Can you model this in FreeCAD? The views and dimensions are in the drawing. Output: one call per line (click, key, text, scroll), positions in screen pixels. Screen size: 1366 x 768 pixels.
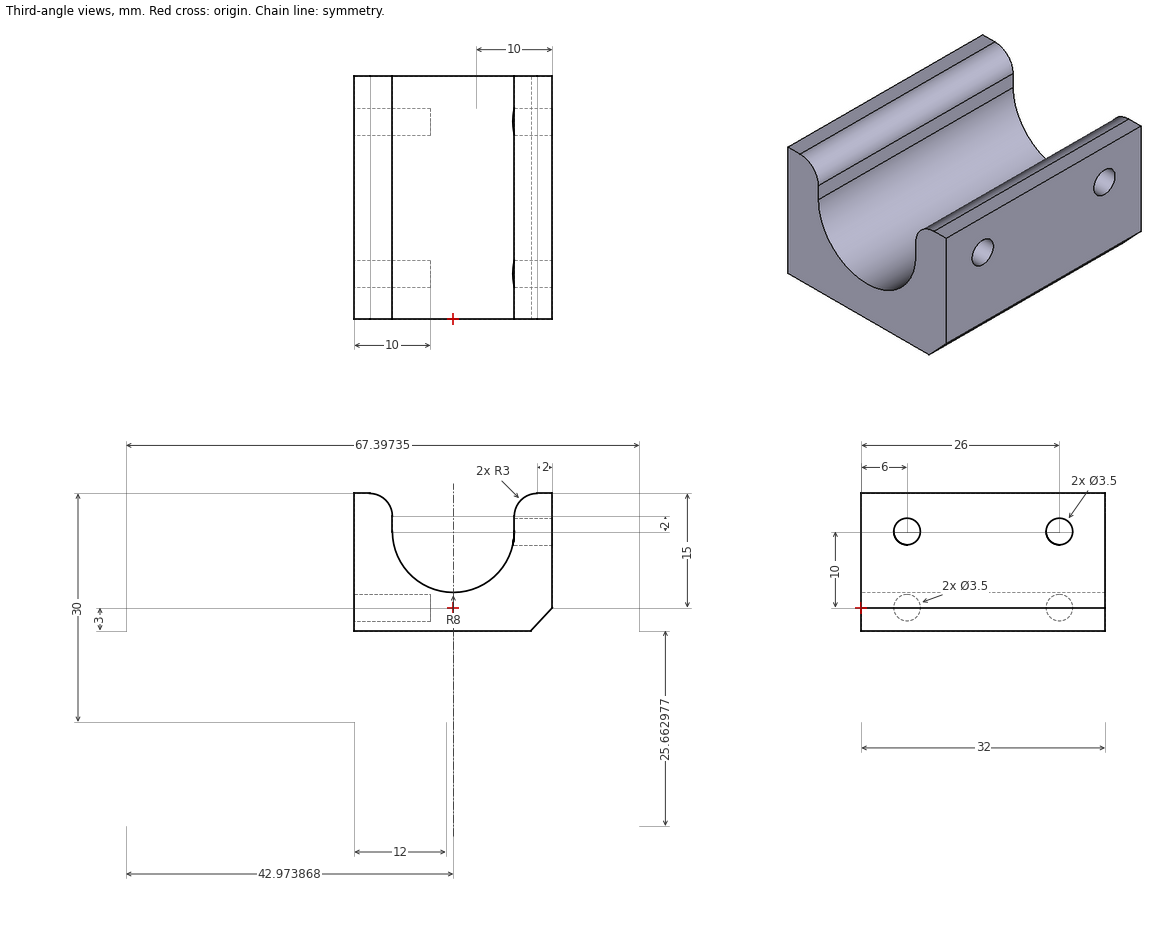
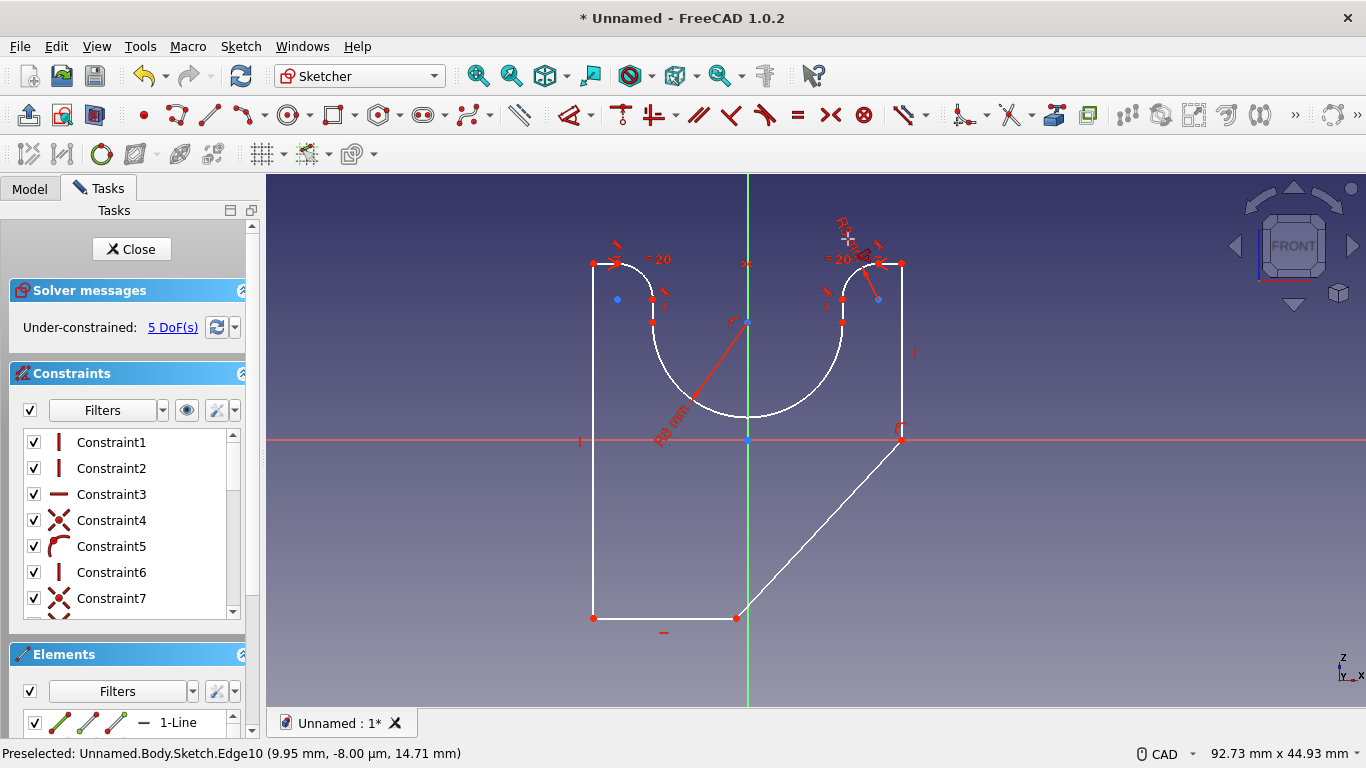
scroll(653, 309, up, 3)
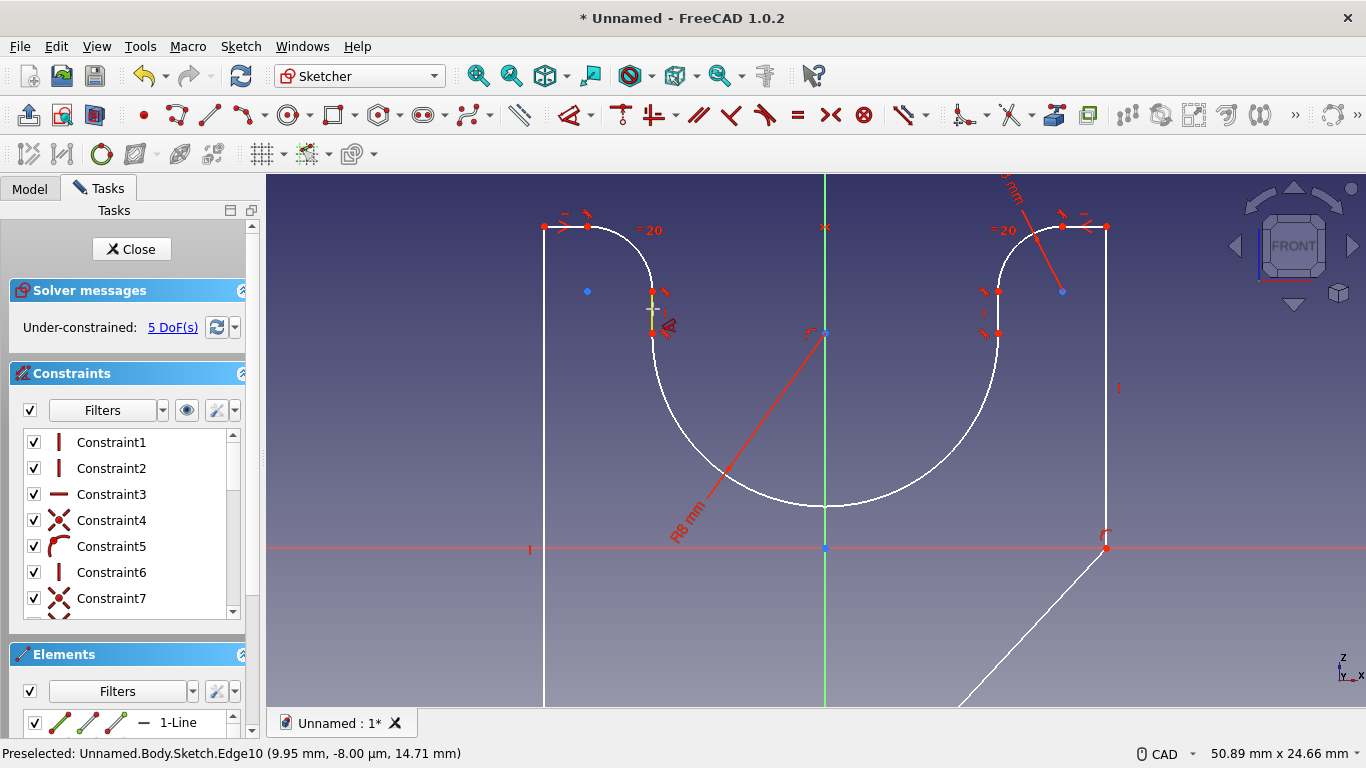
click(652, 308)
click(618, 313)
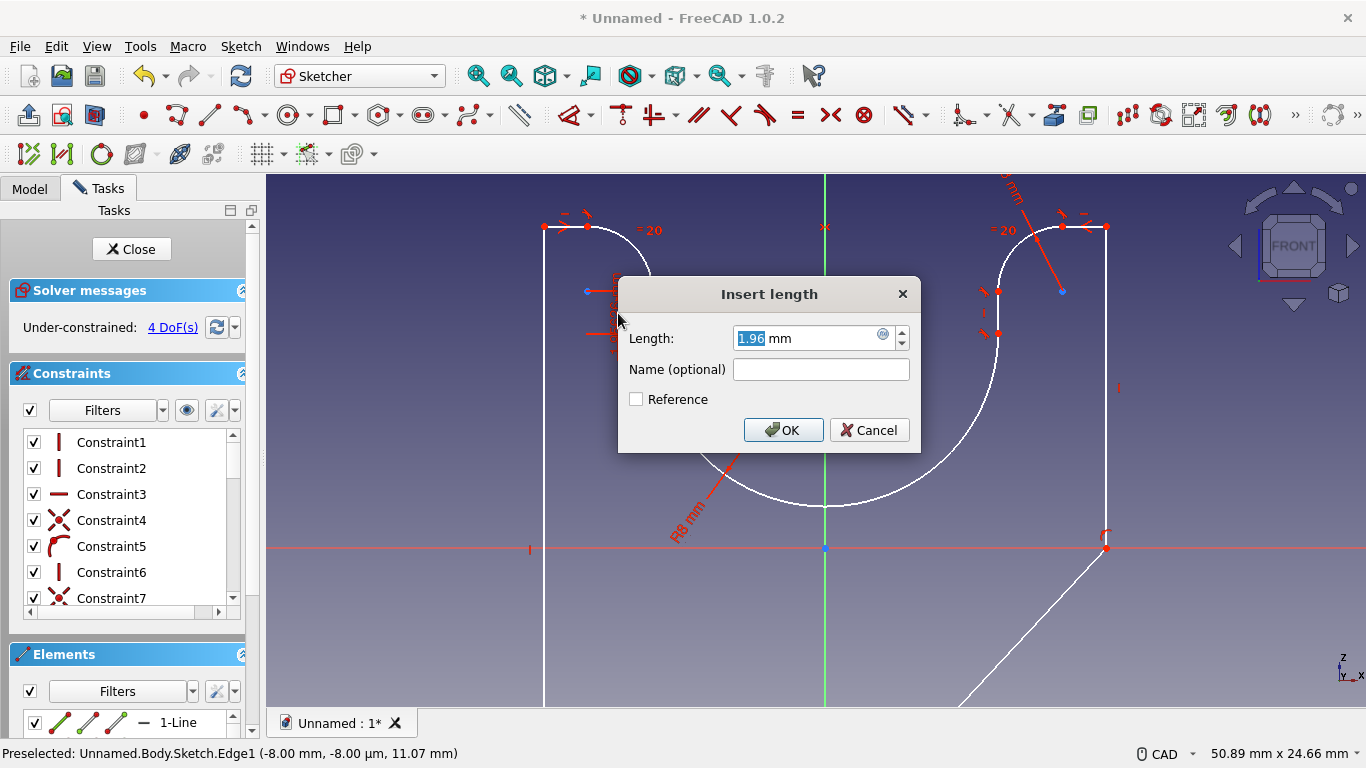
text(2)
key(Return)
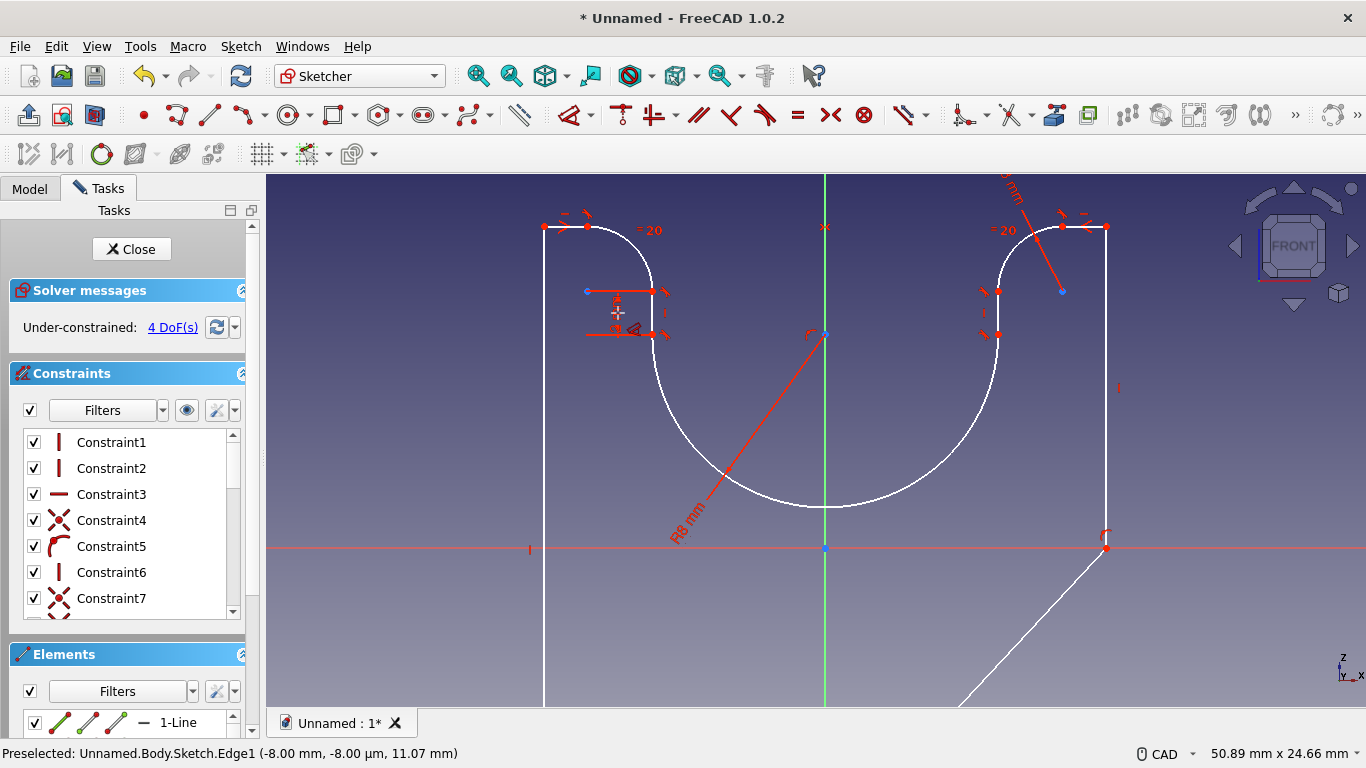
click(1076, 227)
click(1085, 261)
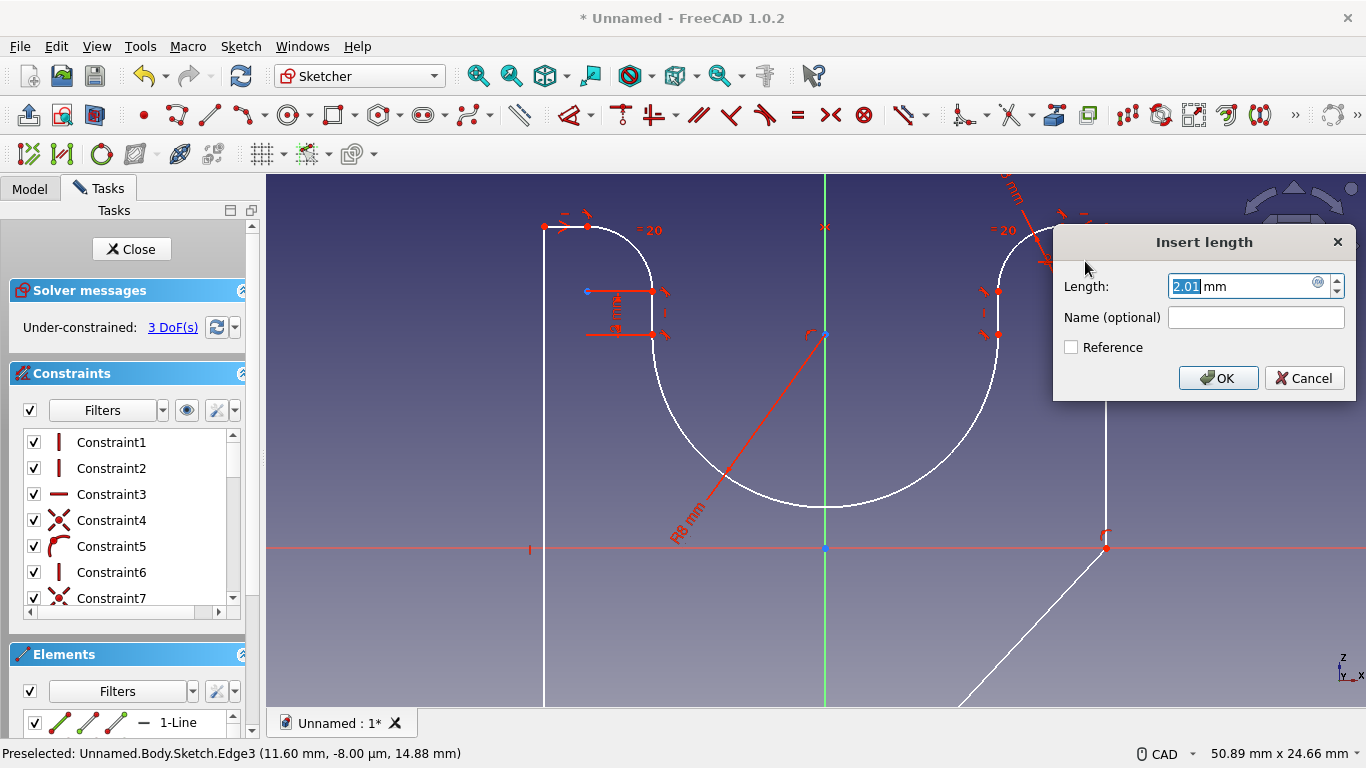
text(2)
key(Return)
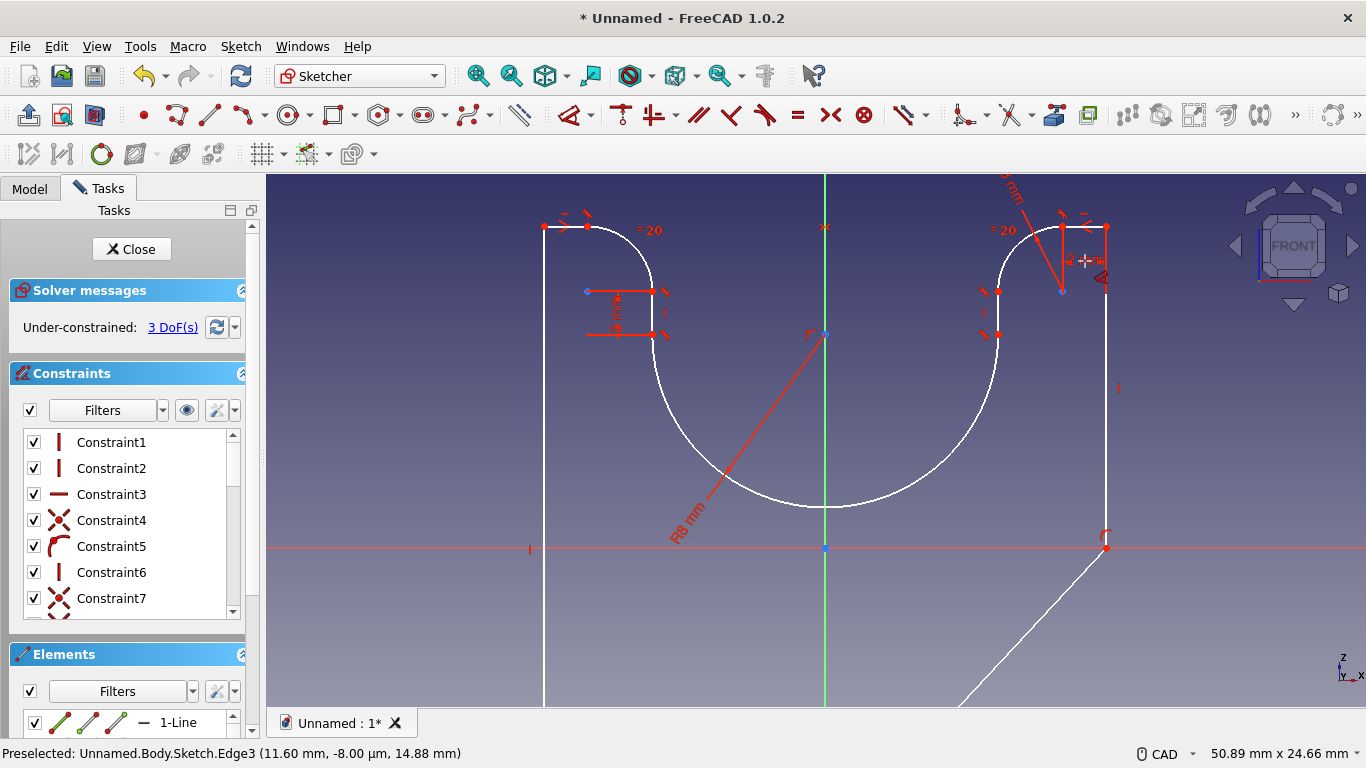
click(1106, 323)
click(1140, 387)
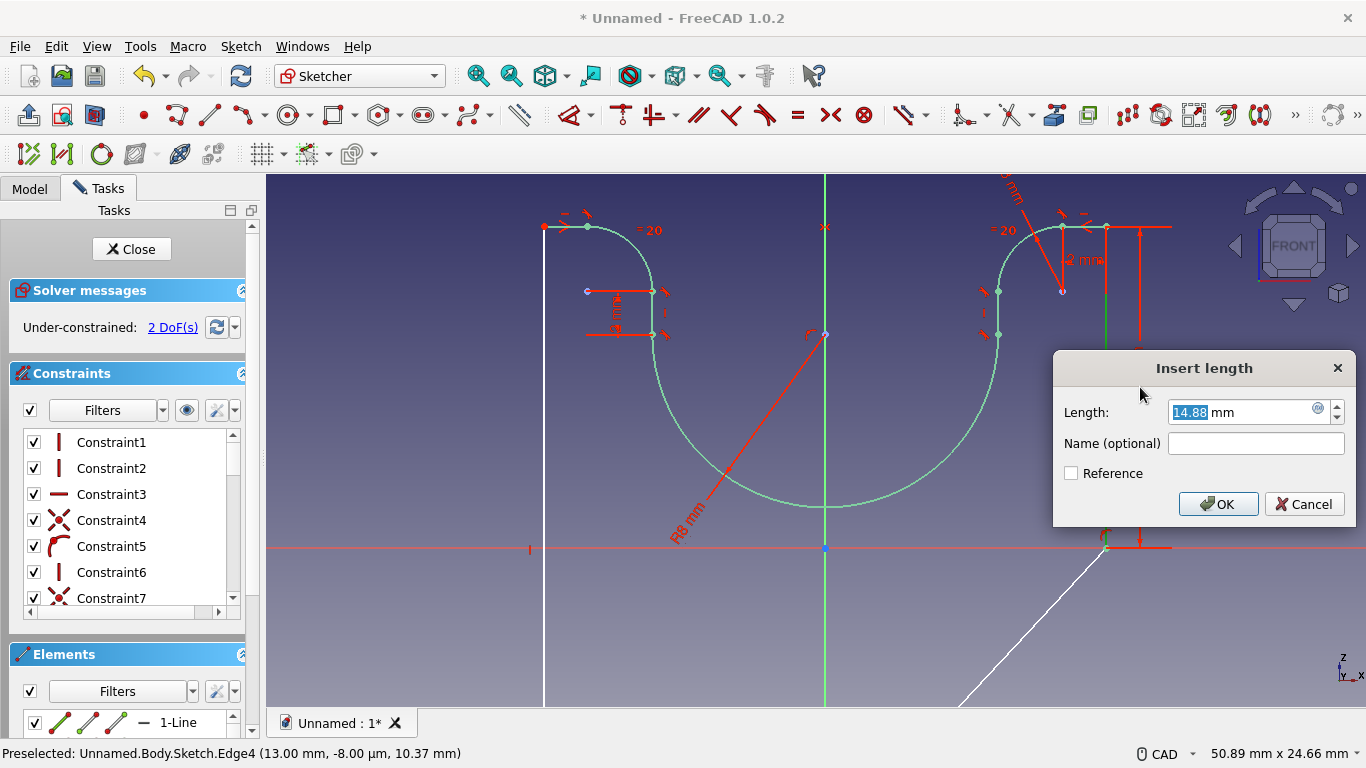
text(15)
key(Return)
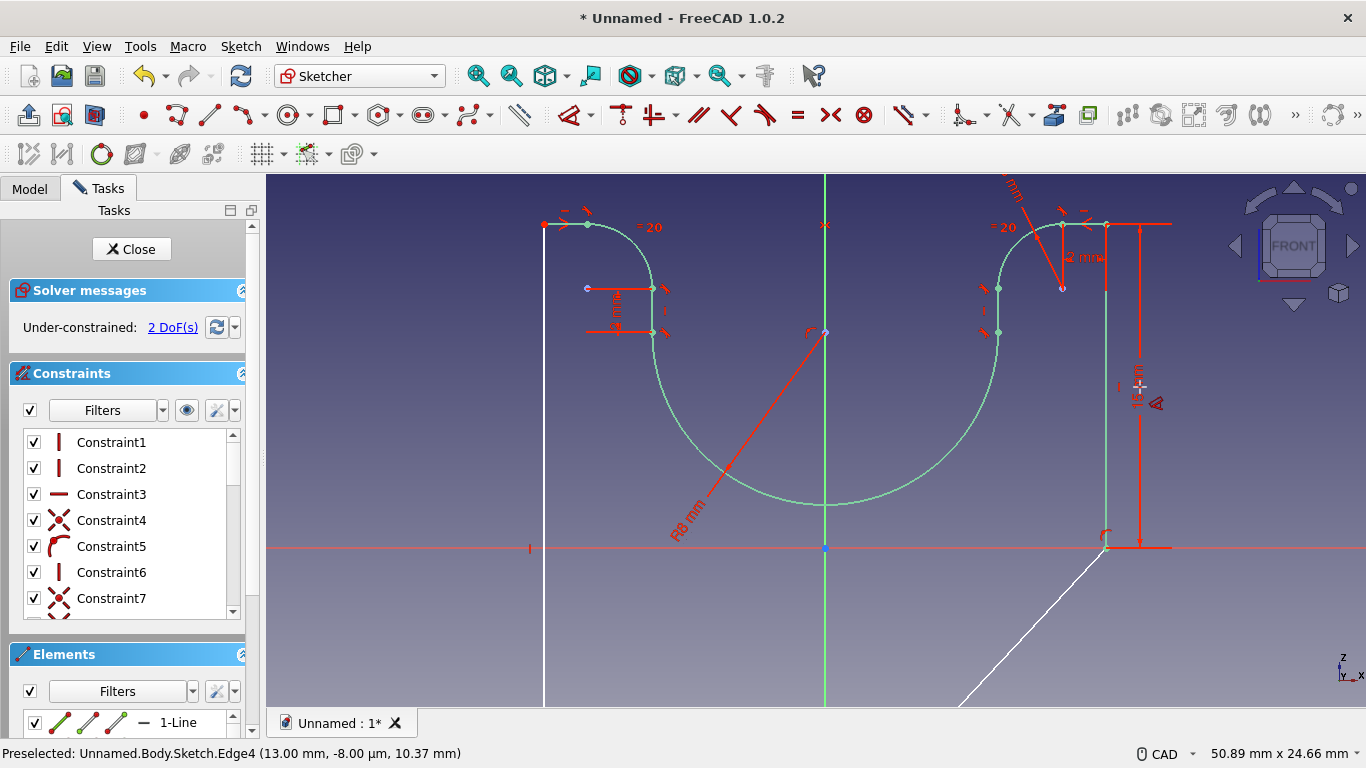
scroll(653, 309, down, 3)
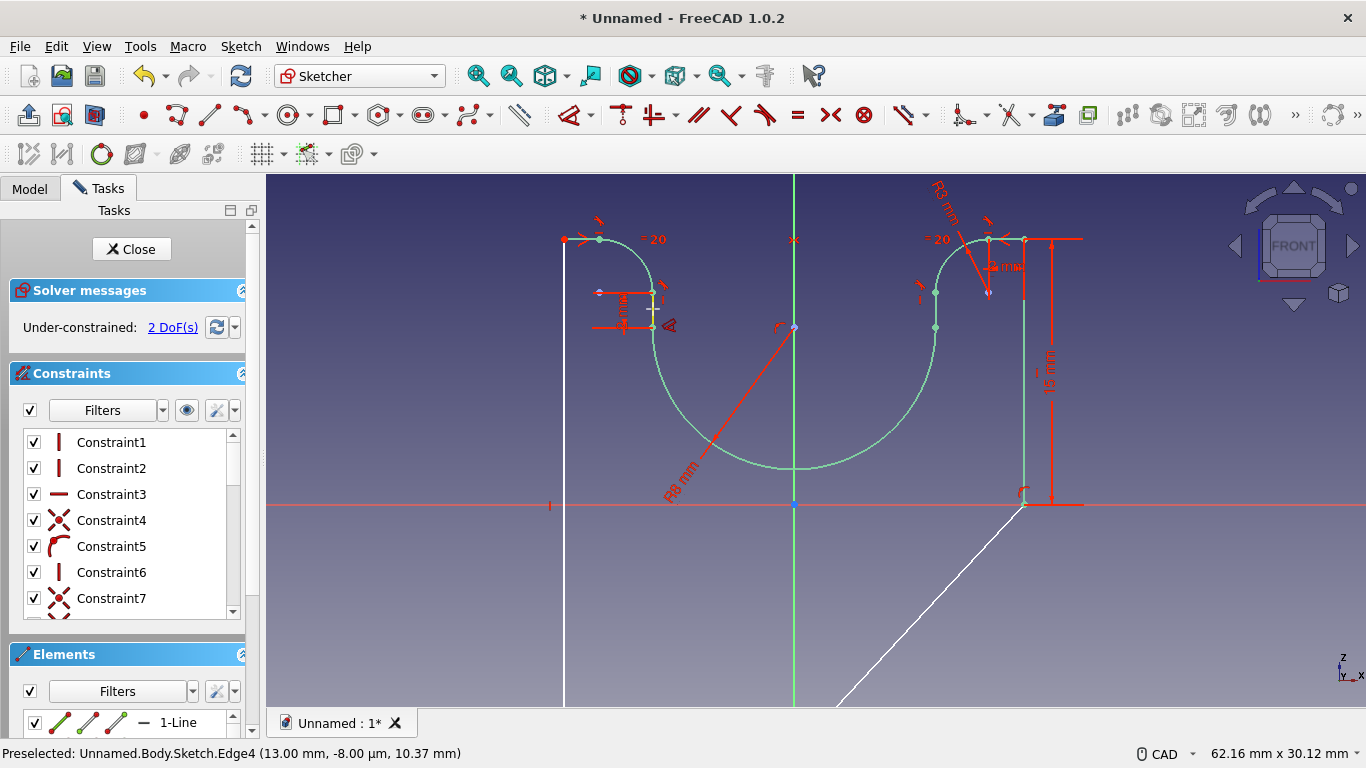
click(693, 619)
click(665, 653)